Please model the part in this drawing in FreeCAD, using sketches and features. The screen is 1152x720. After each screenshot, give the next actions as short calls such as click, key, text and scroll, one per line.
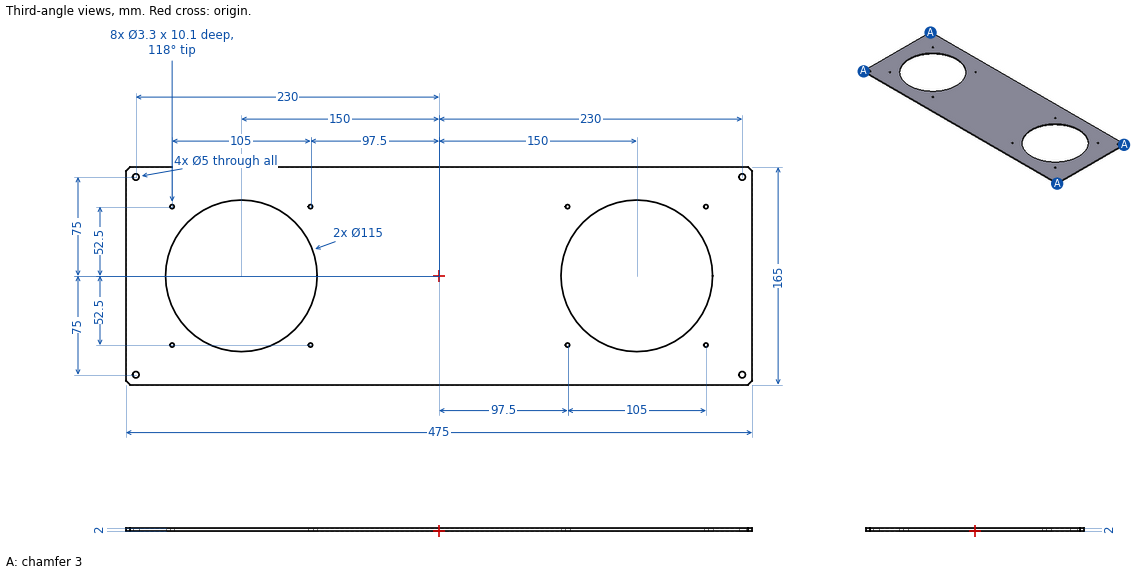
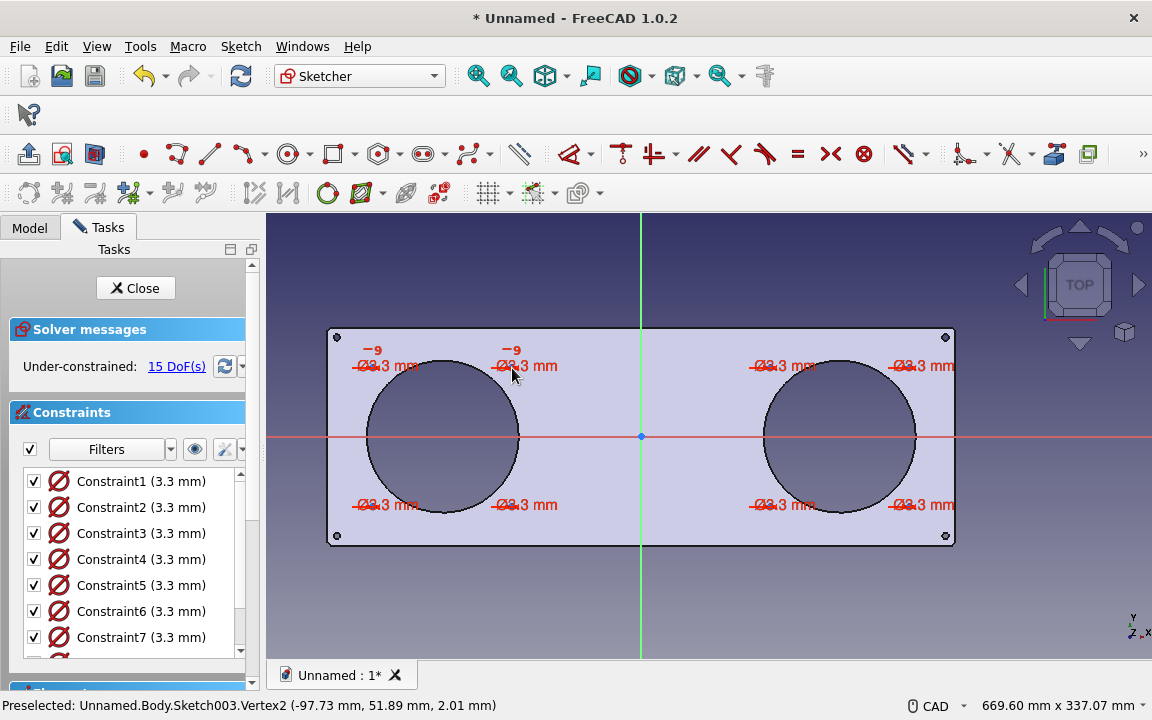
click(512, 368)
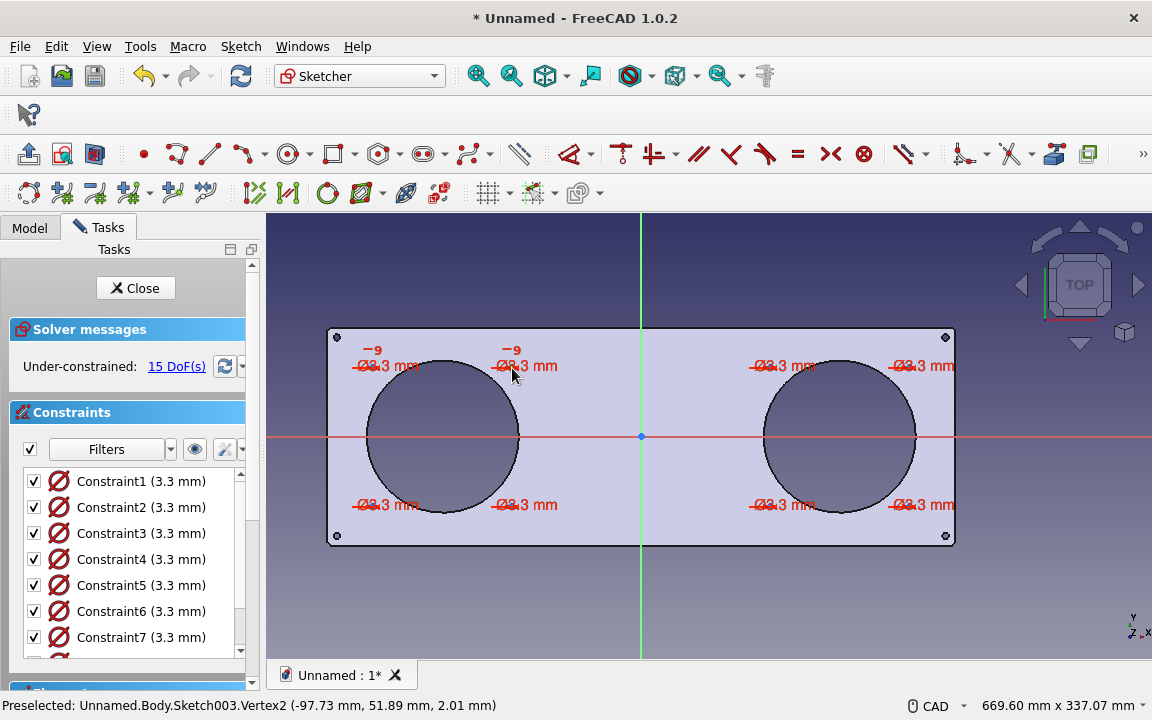
click(512, 507)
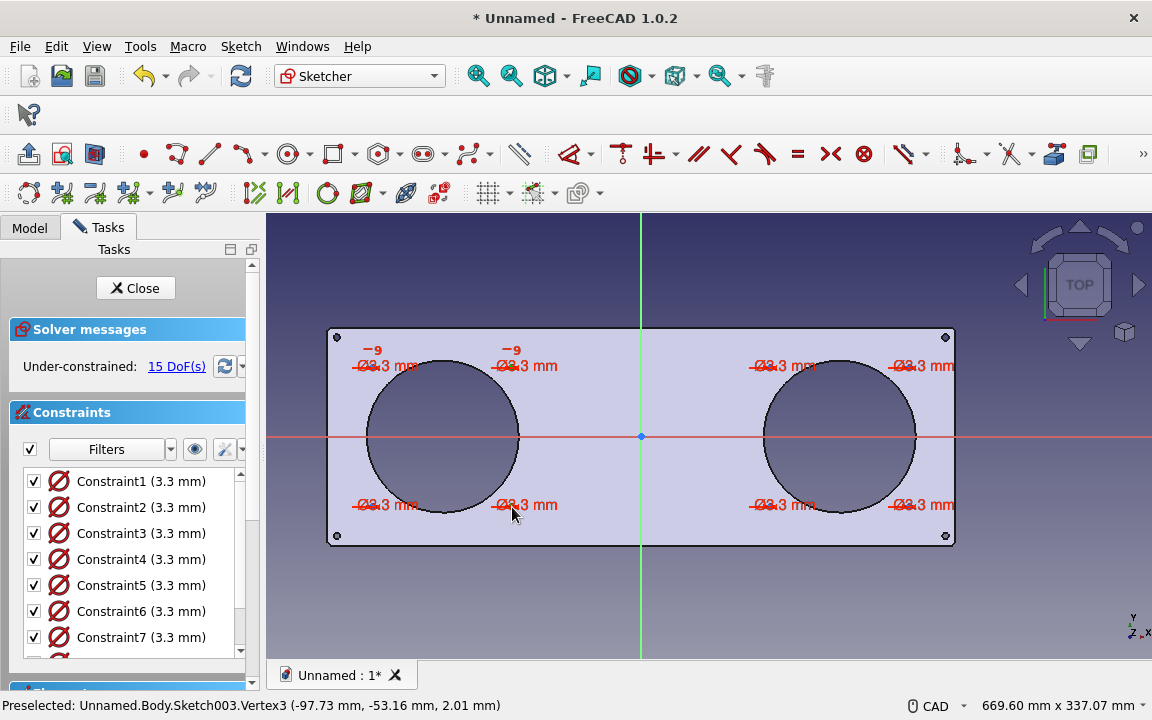
key(v)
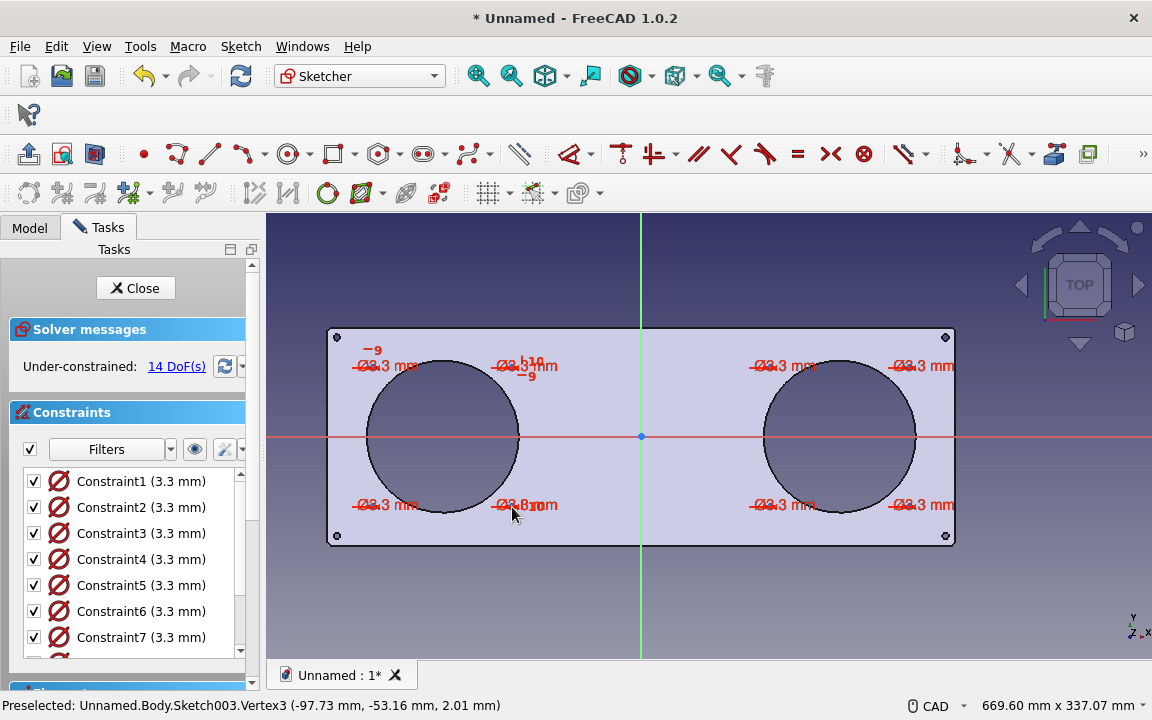
click(373, 368)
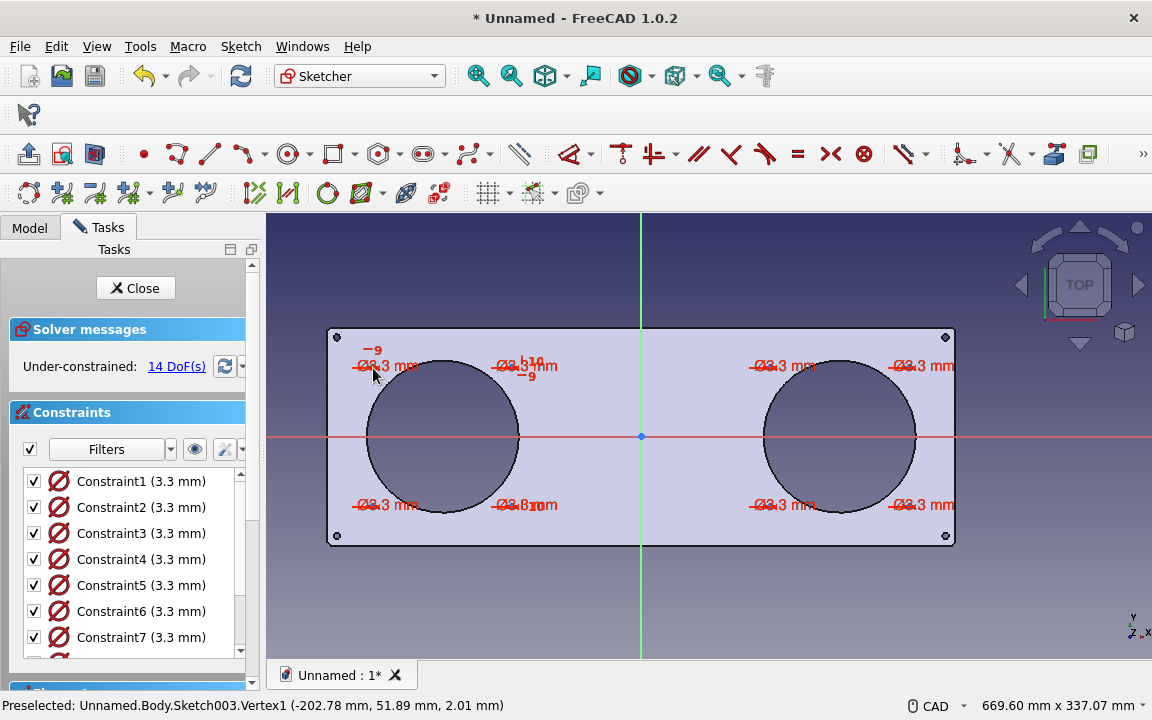
click(373, 507)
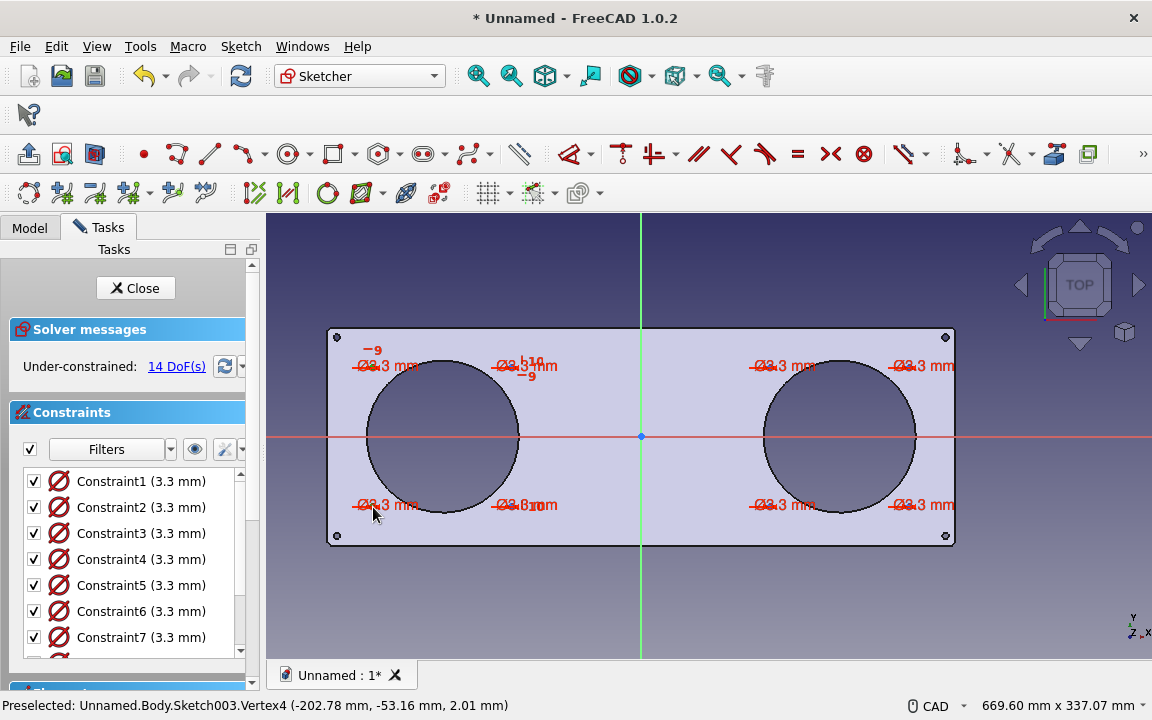
key(v)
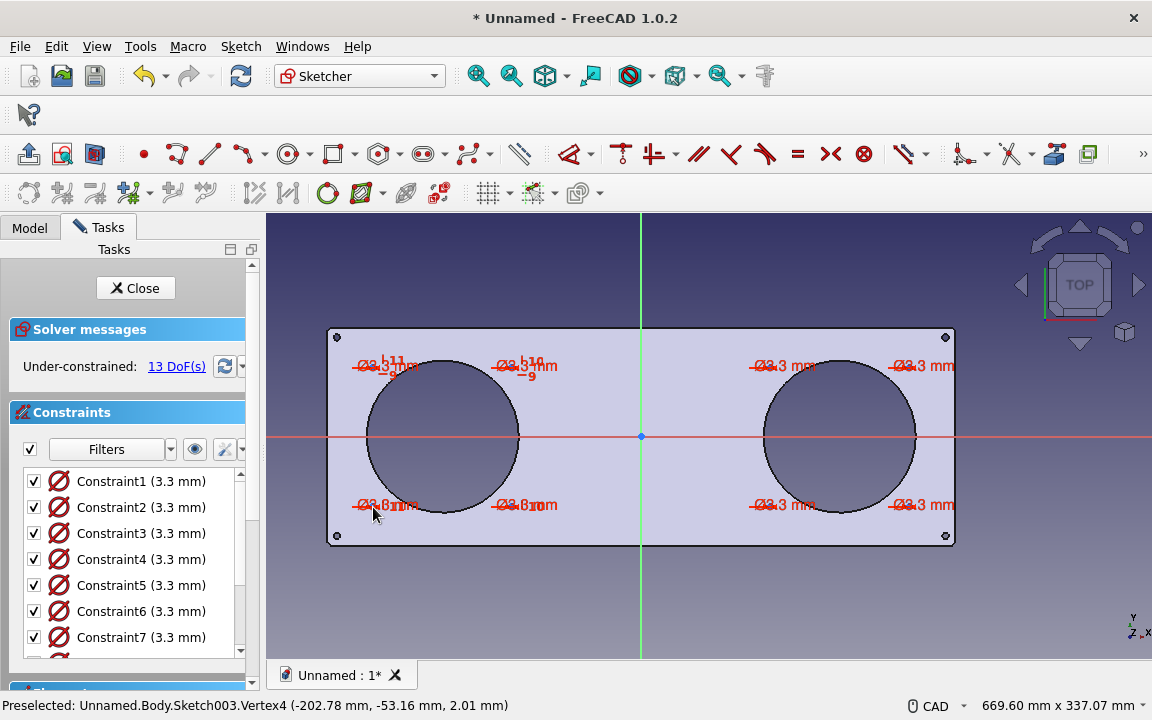
click(512, 507)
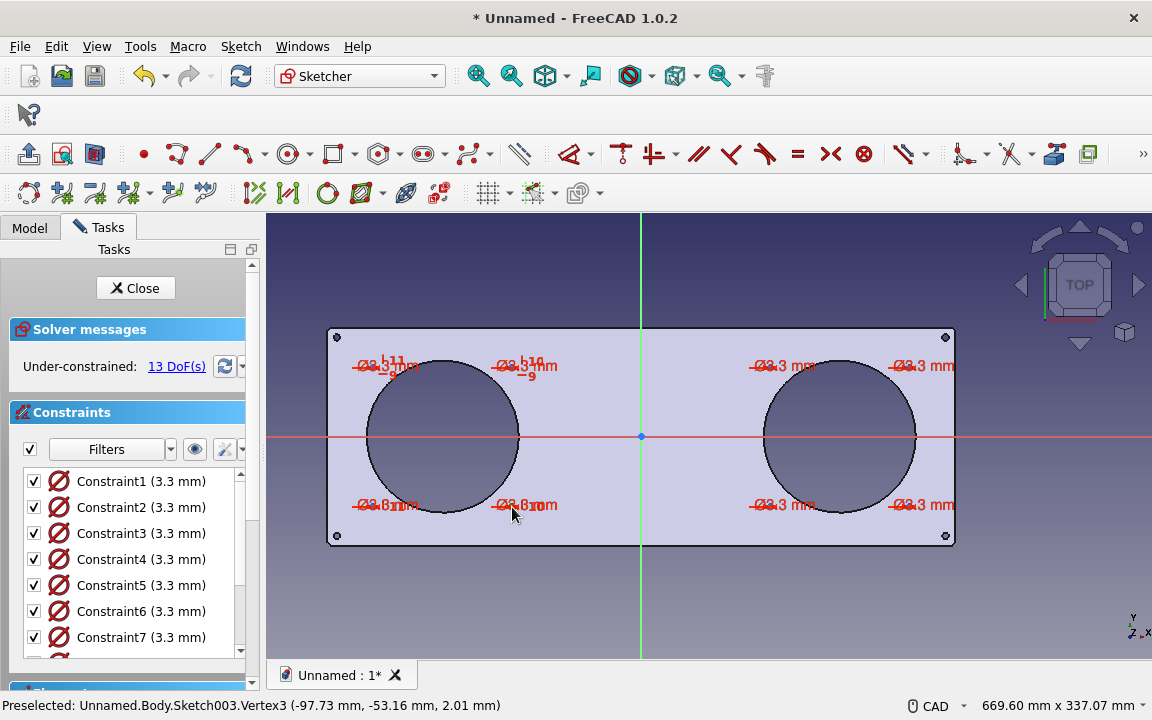
click(373, 507)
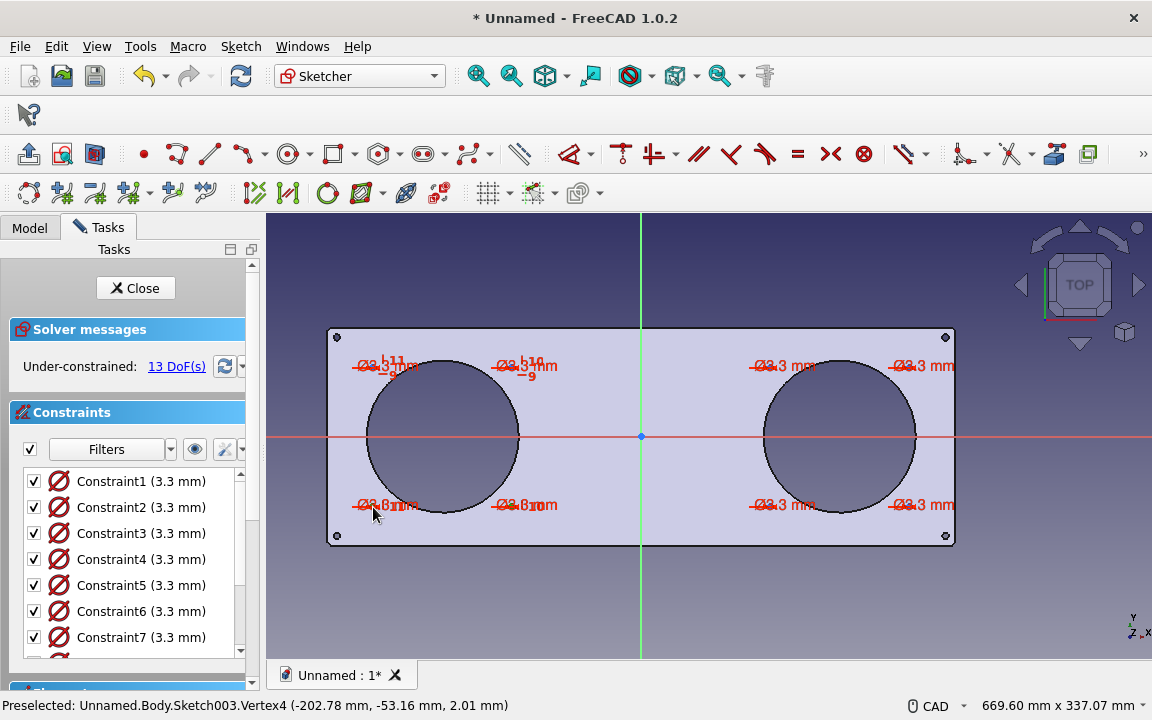
key(h)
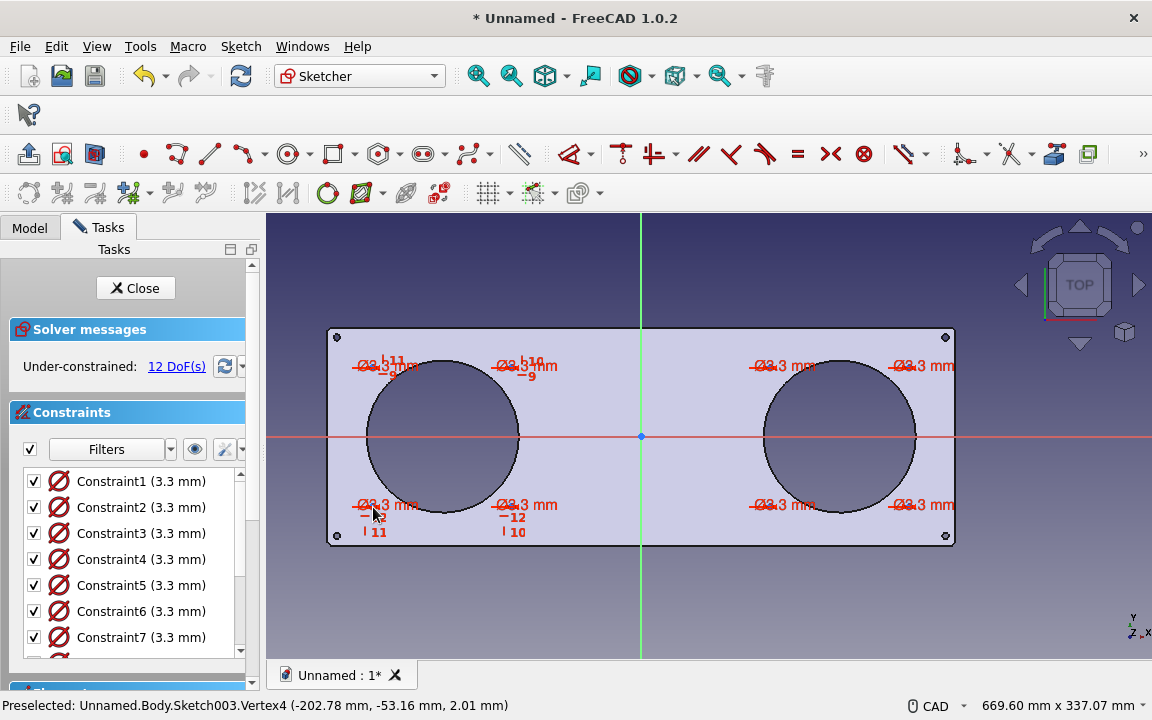
click(512, 507)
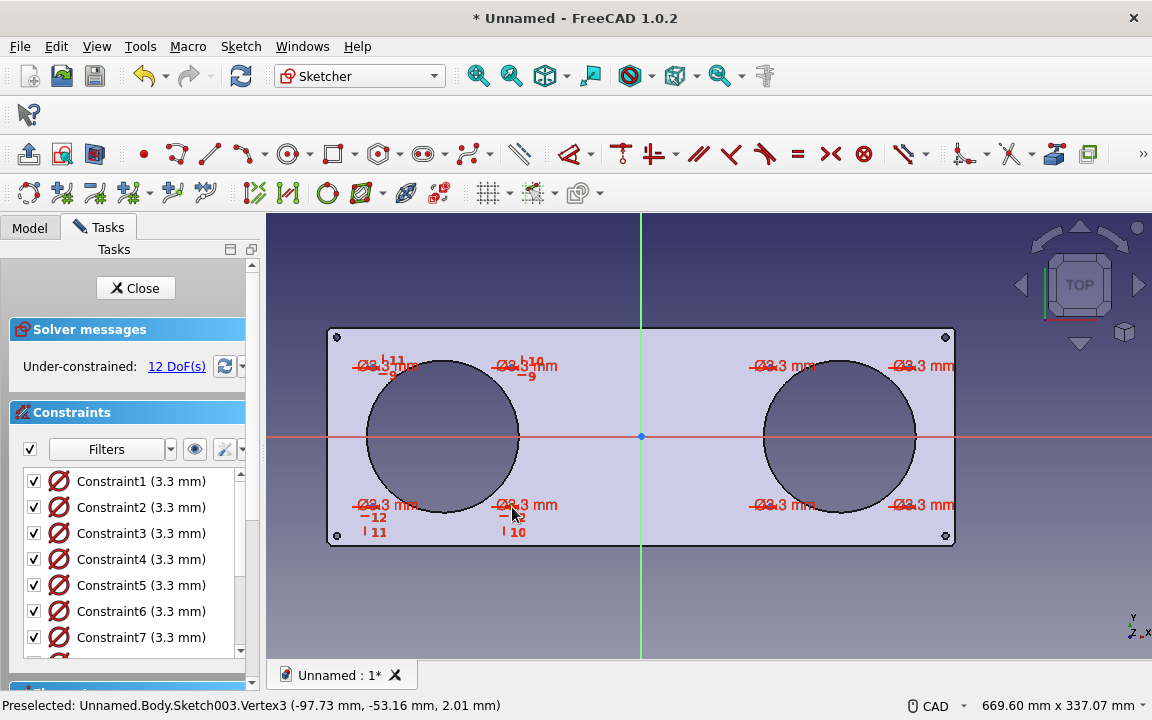
click(770, 507)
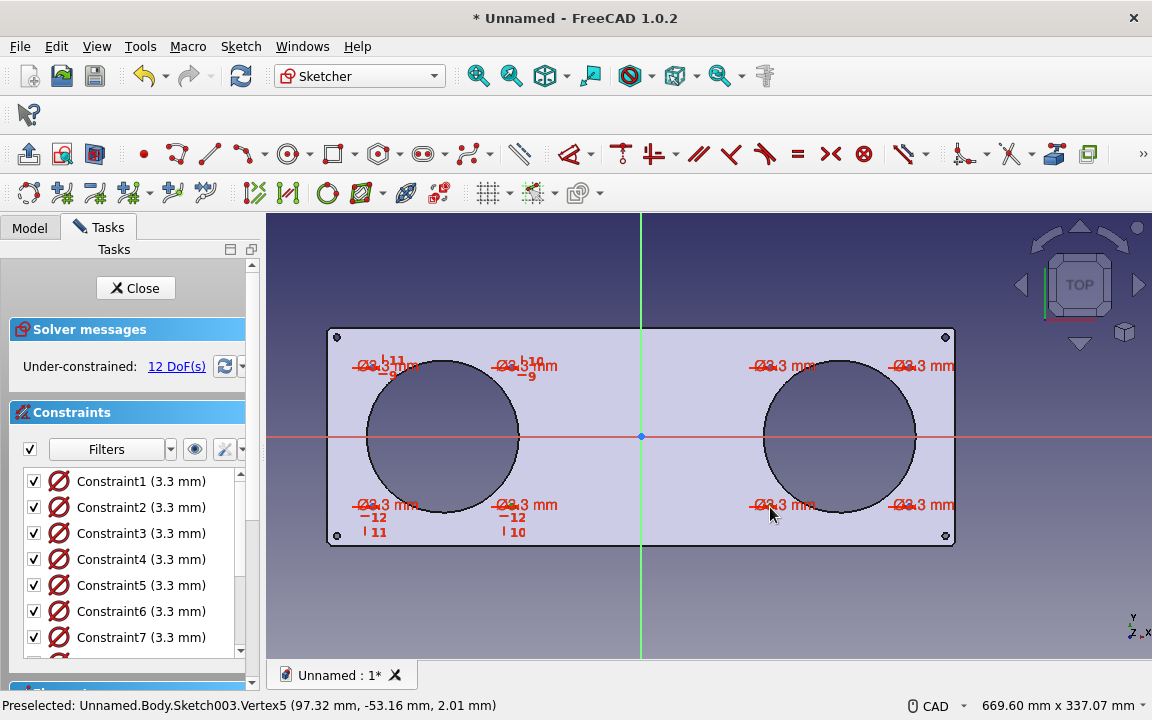
click(676, 154)